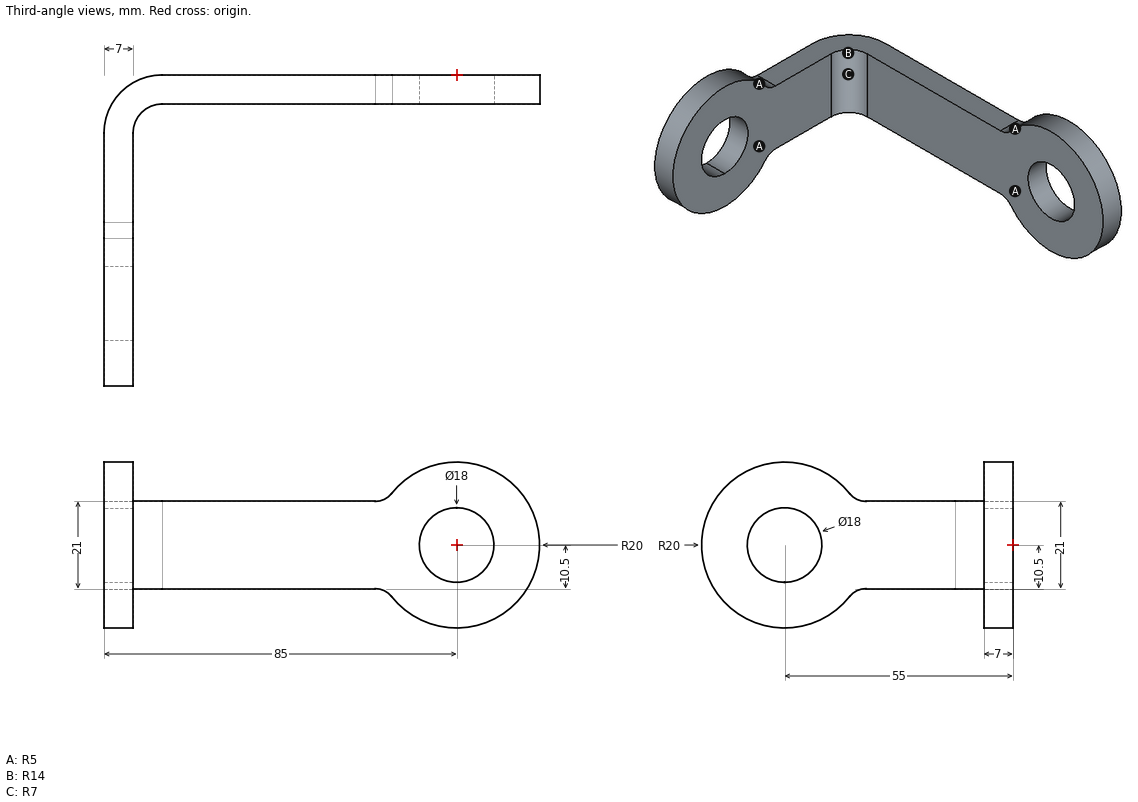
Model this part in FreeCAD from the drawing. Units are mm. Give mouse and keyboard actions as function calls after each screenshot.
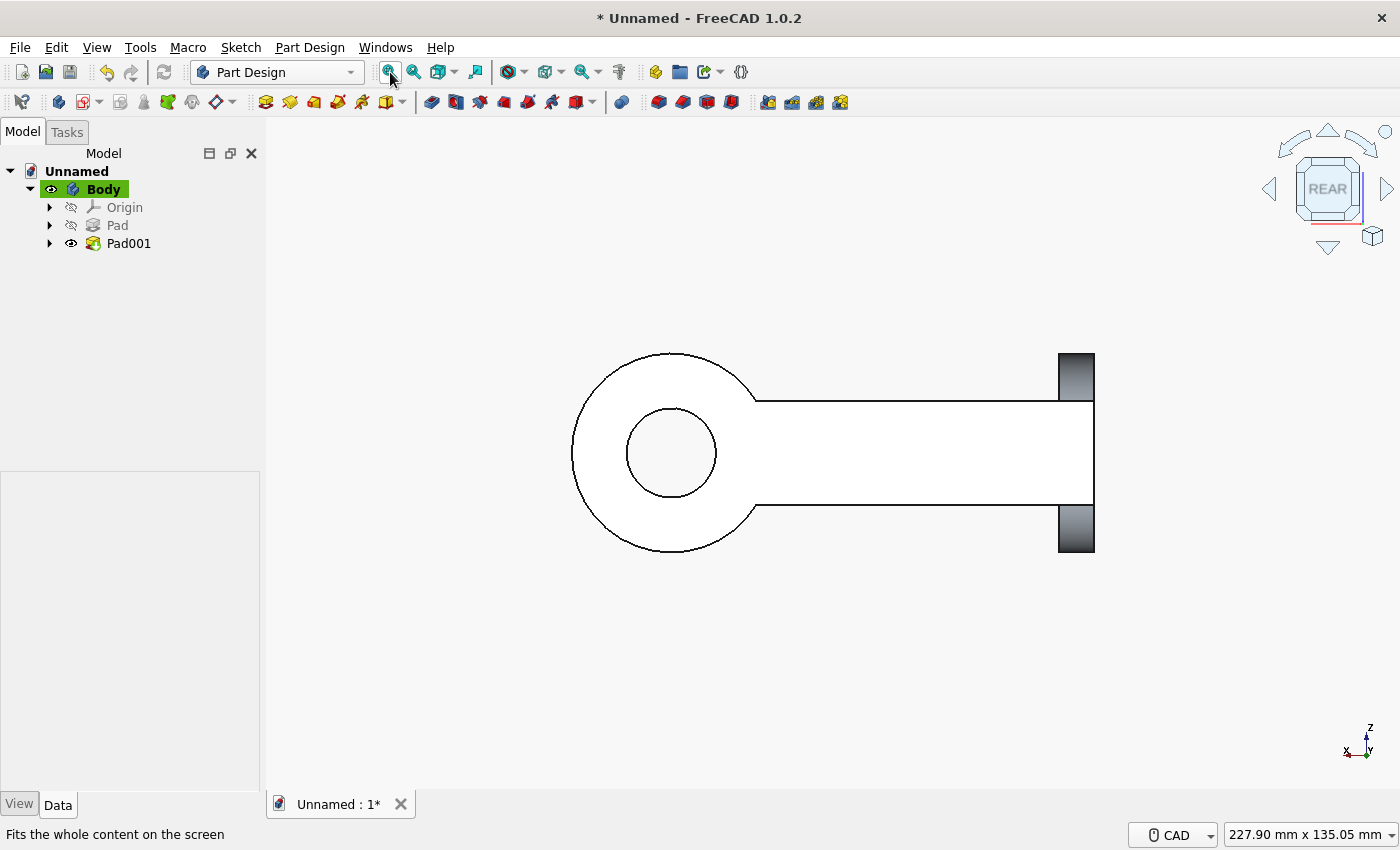
key(6)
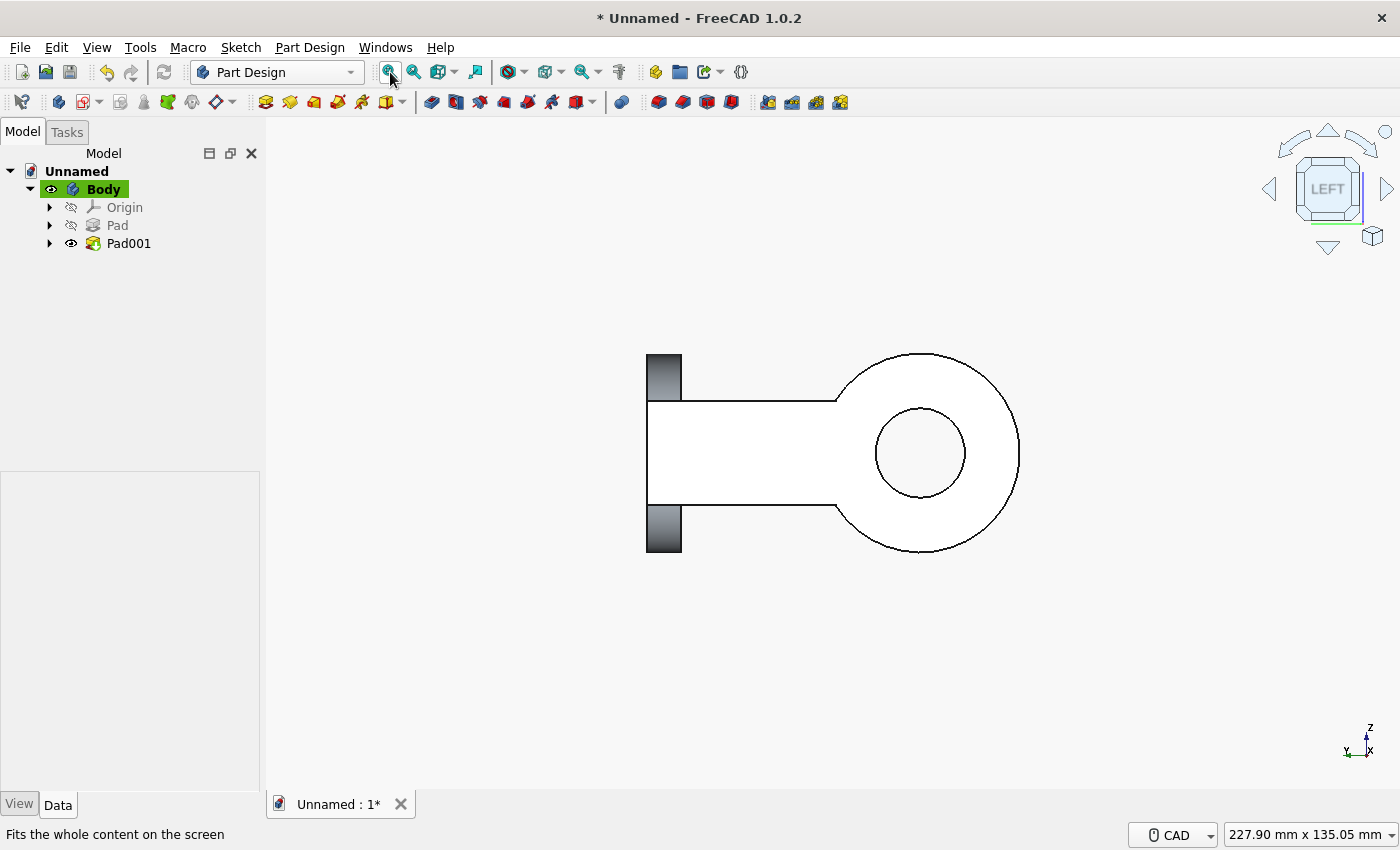
click(390, 72)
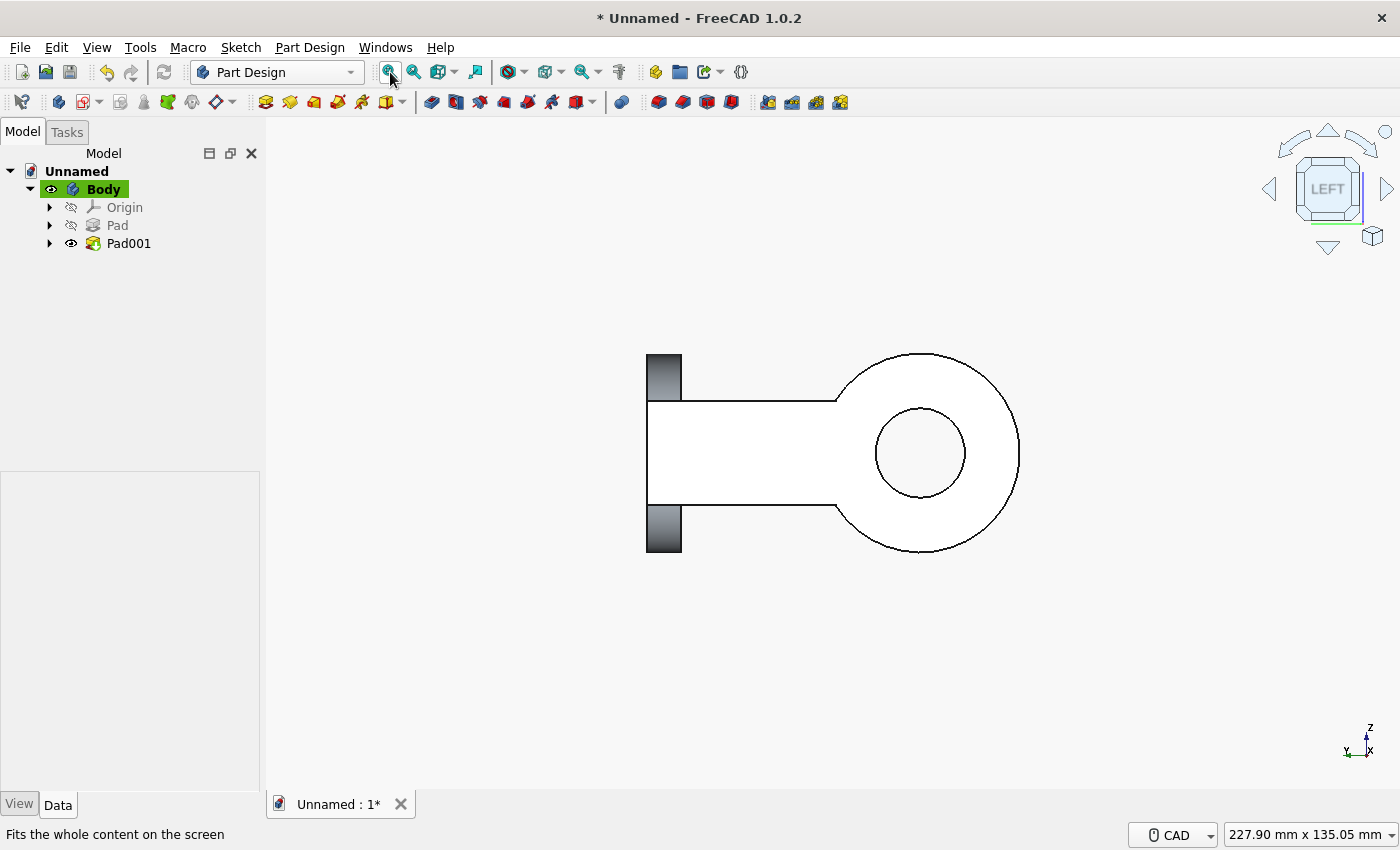
key(v)
key(3)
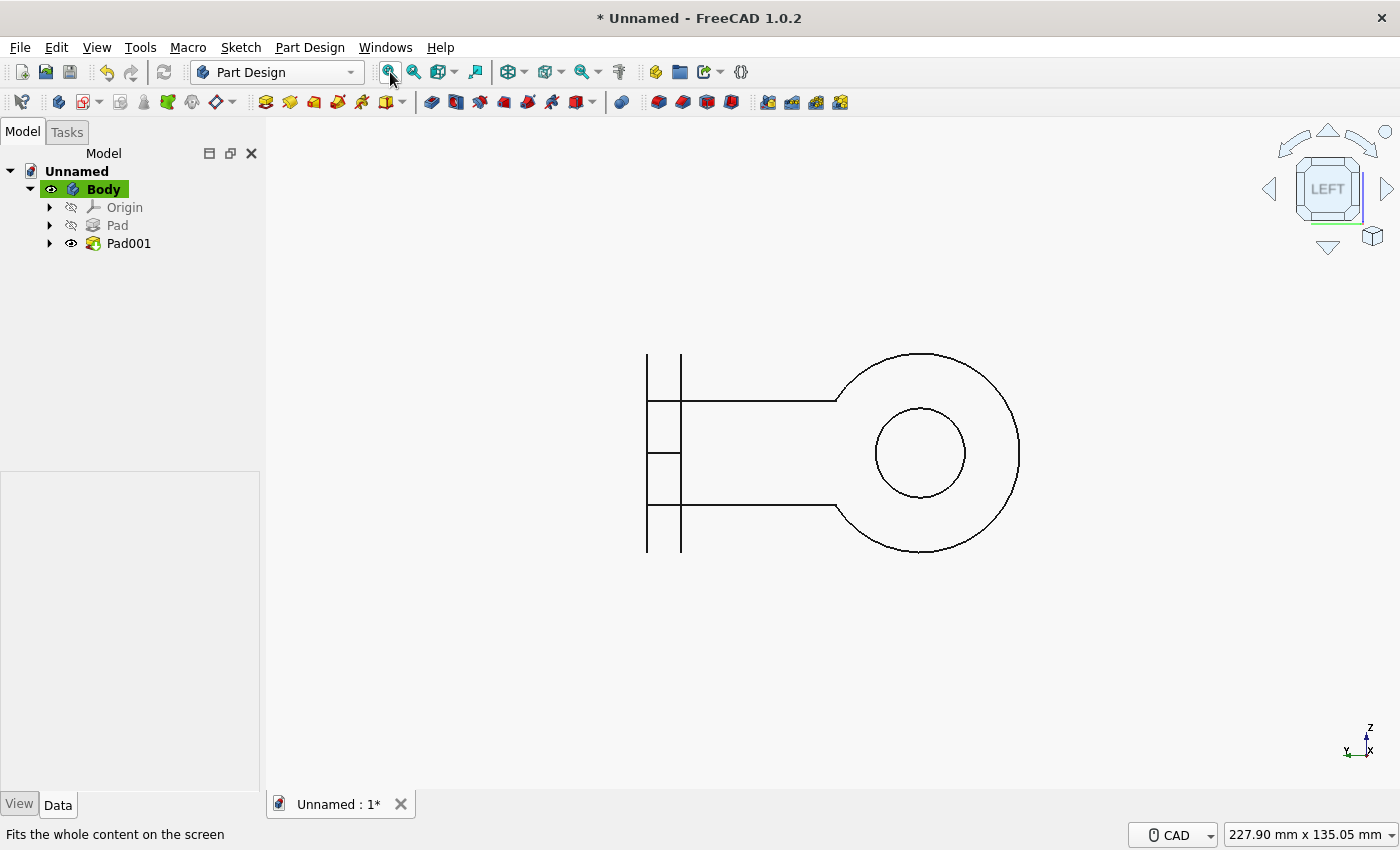
key(0)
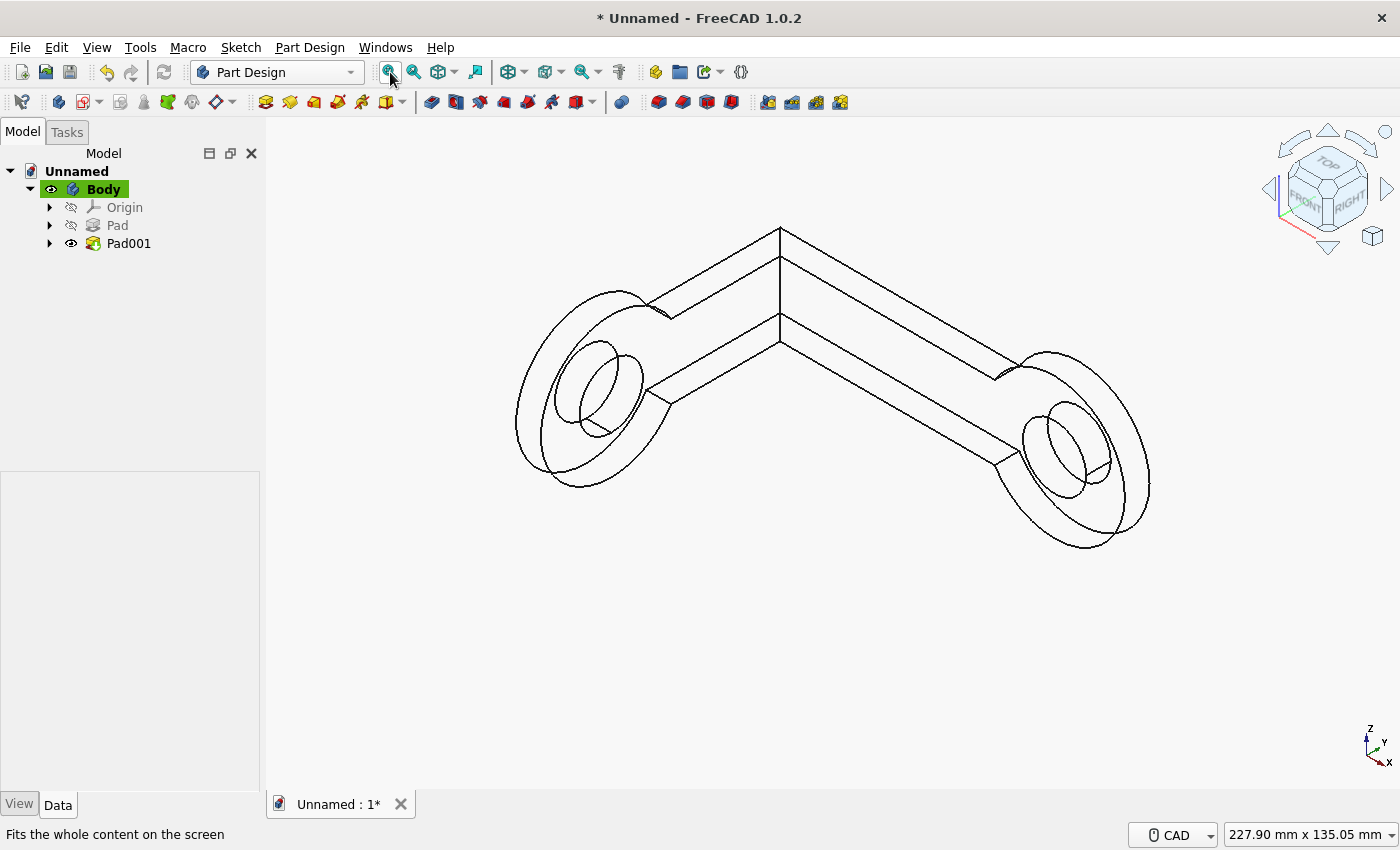
click(659, 396)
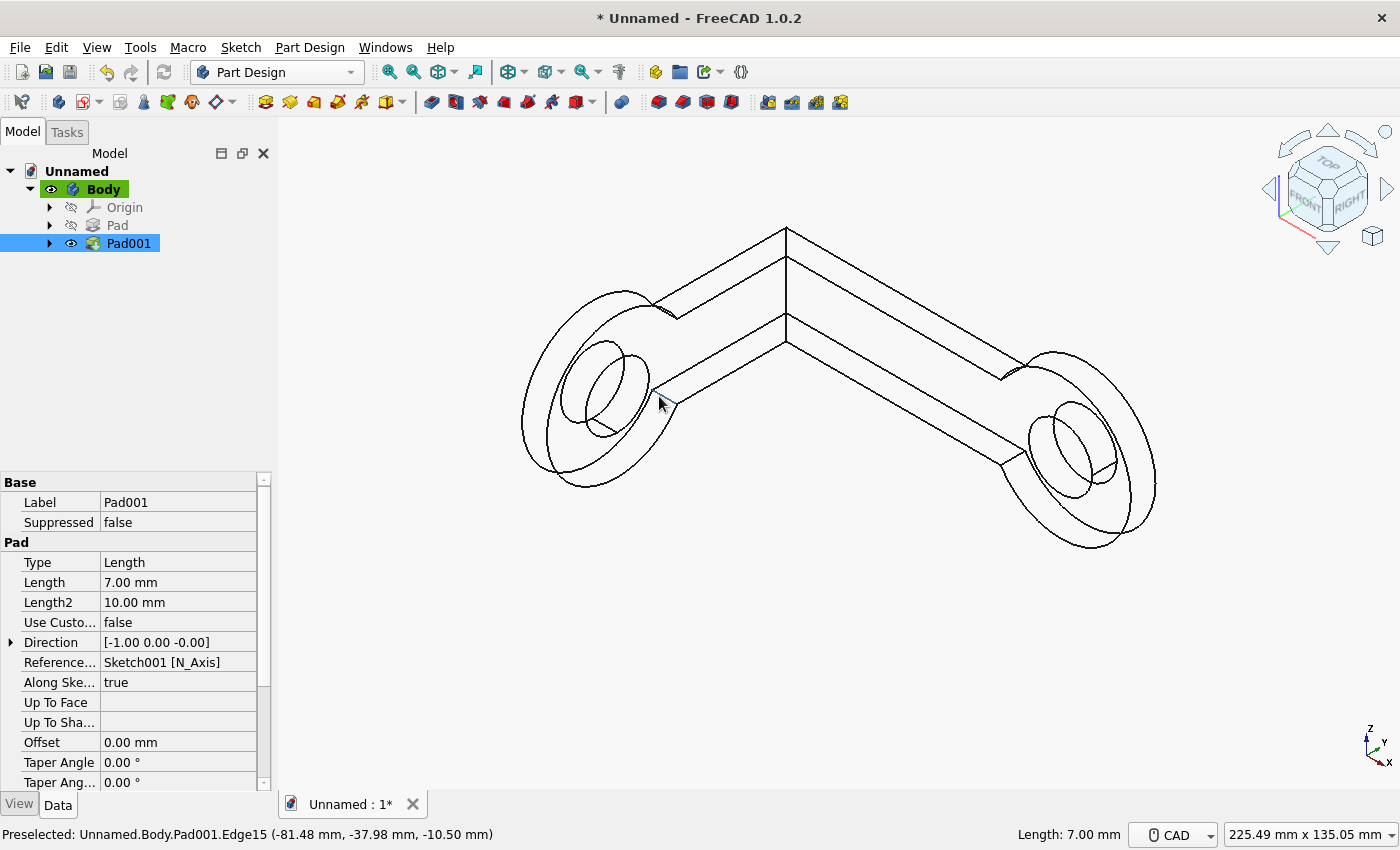
click(1013, 457, ctrl)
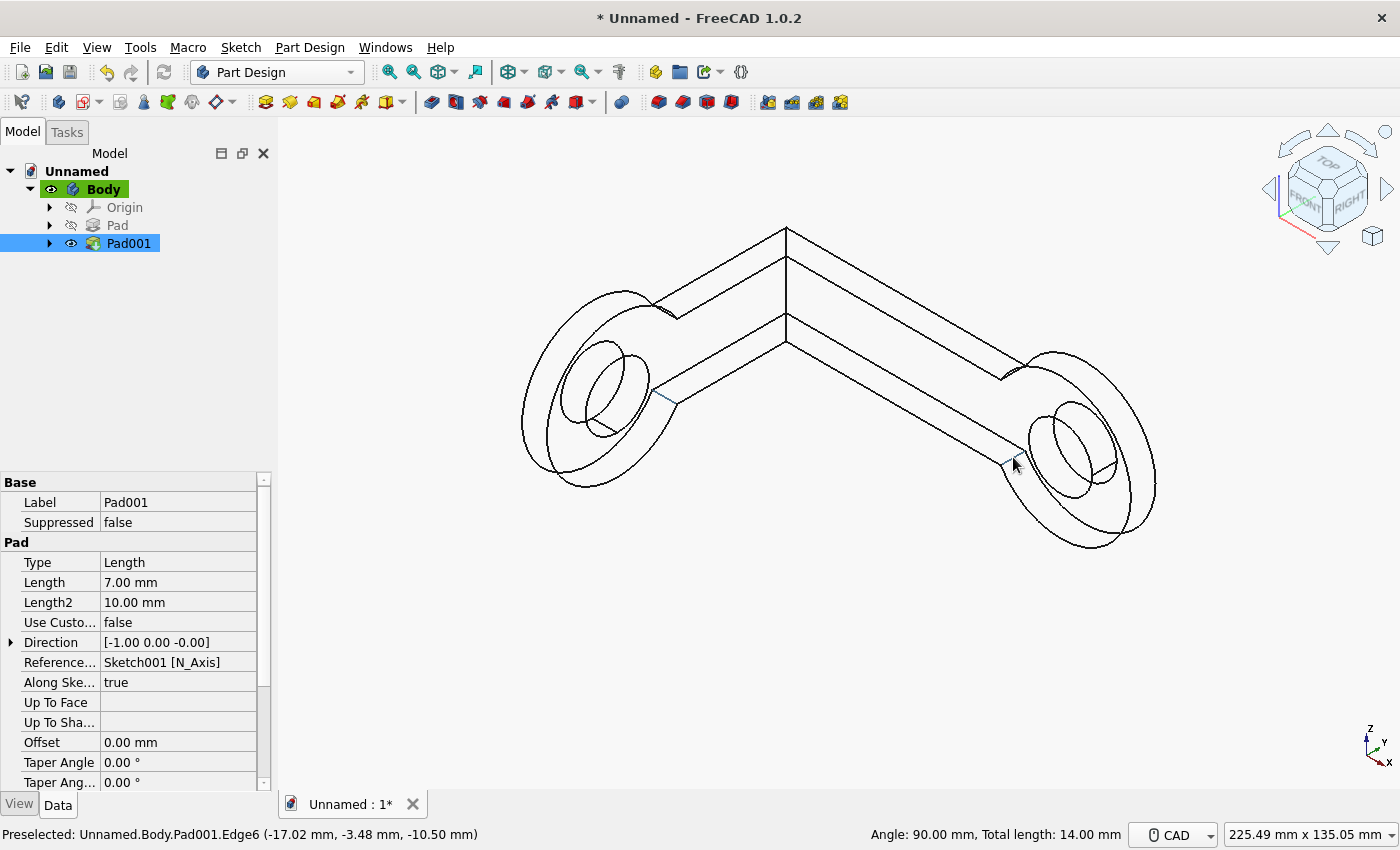
scroll(665, 311, up, 6)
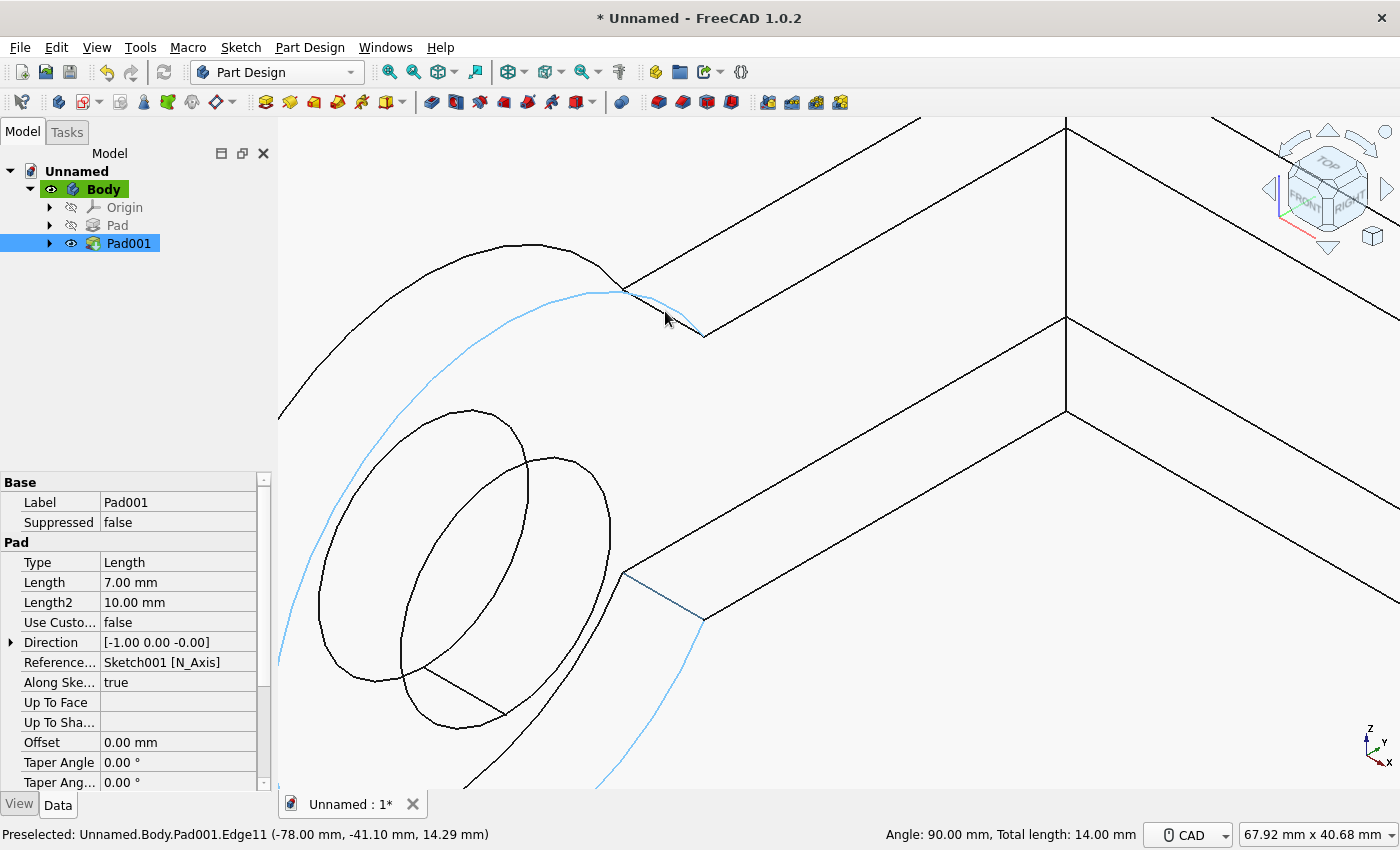
click(664, 312, ctrl)